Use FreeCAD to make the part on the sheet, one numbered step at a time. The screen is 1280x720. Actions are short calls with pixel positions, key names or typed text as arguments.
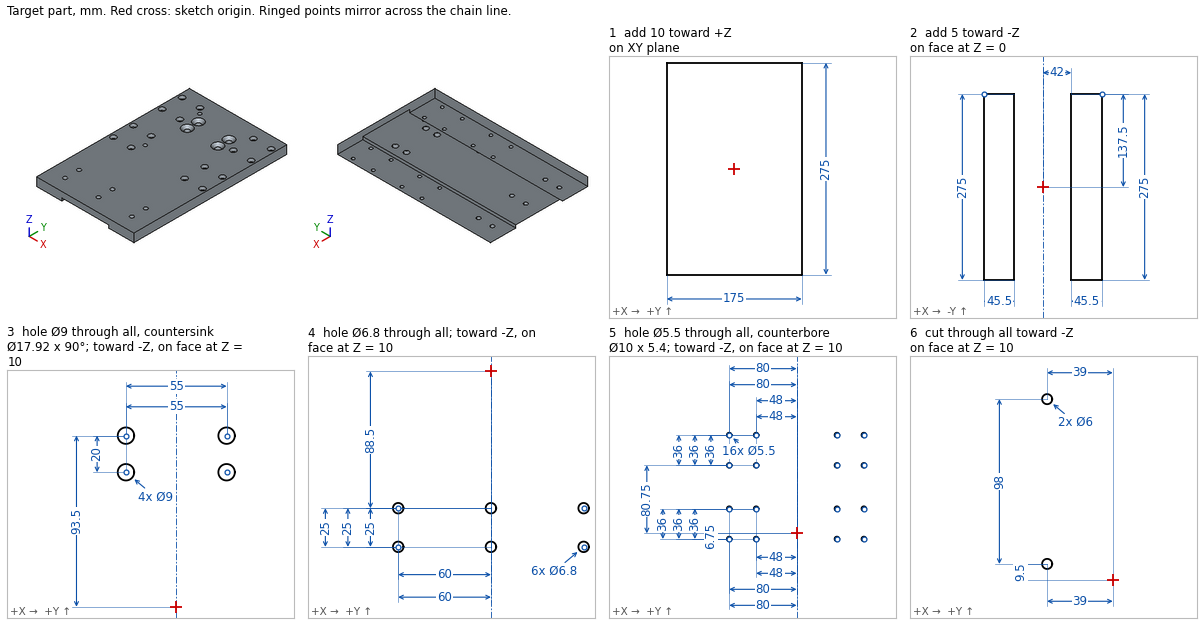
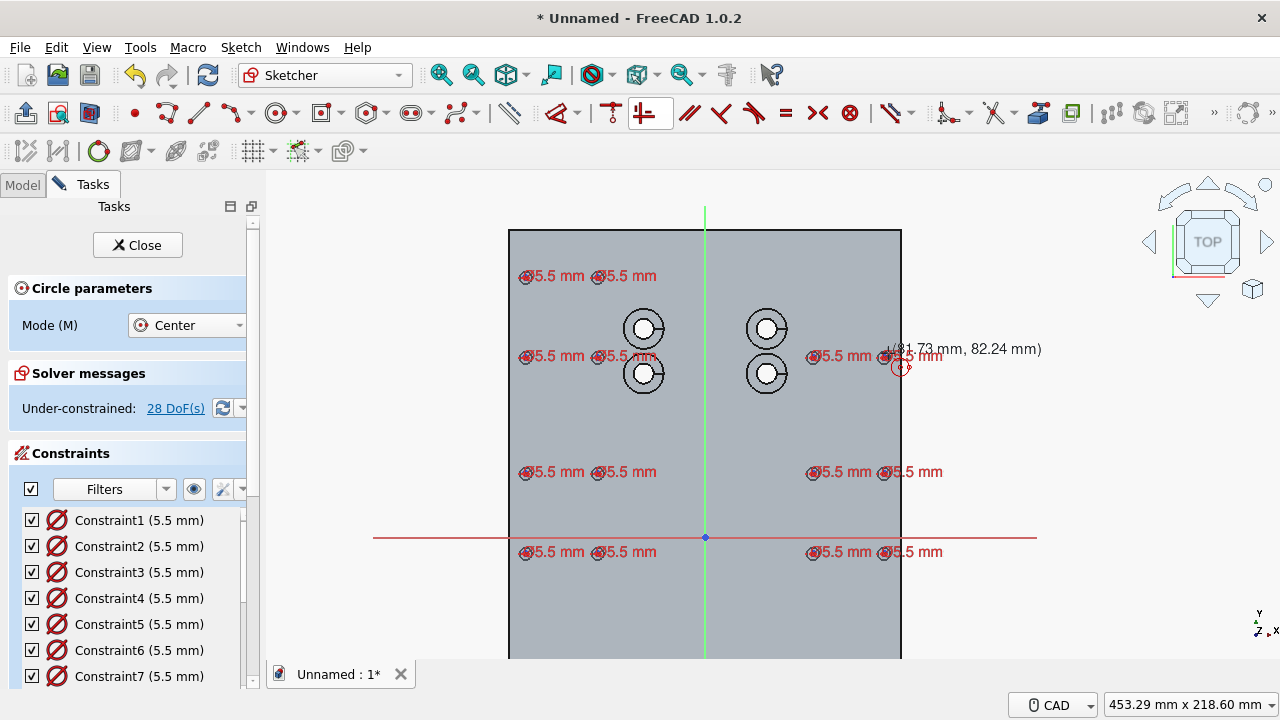
scroll(813, 277, up, 7)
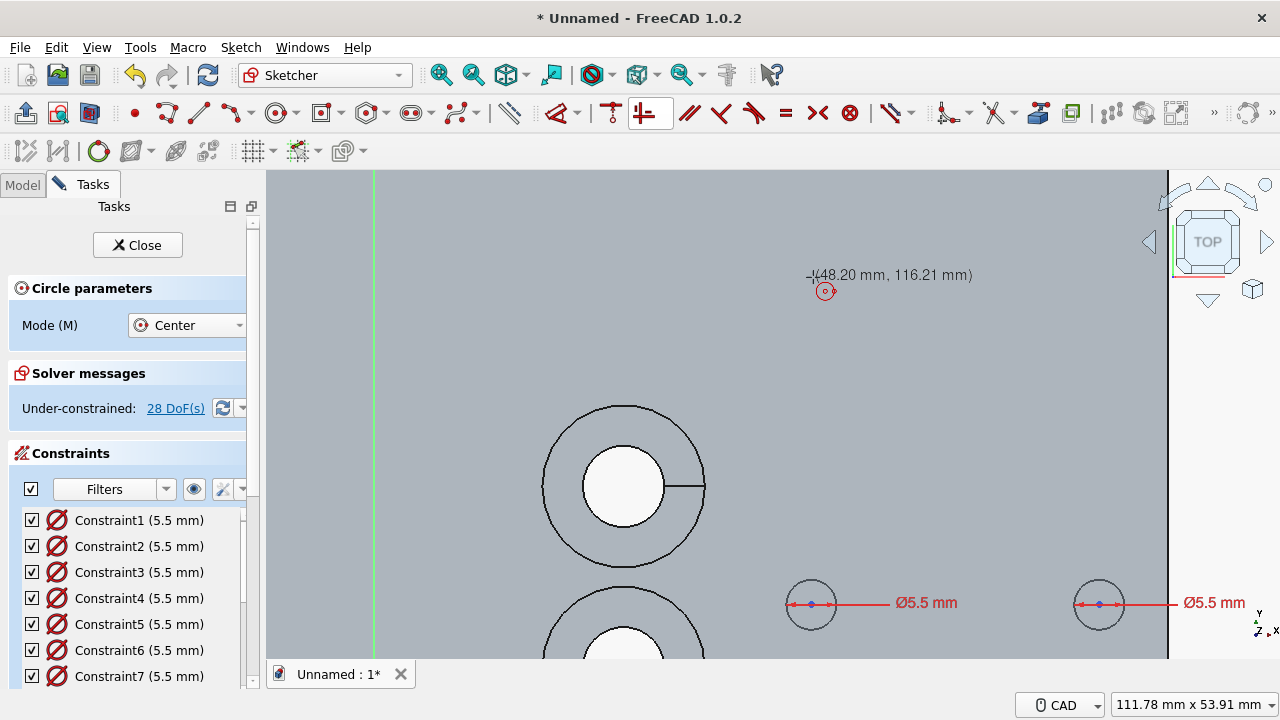
scroll(813, 277, down, 7)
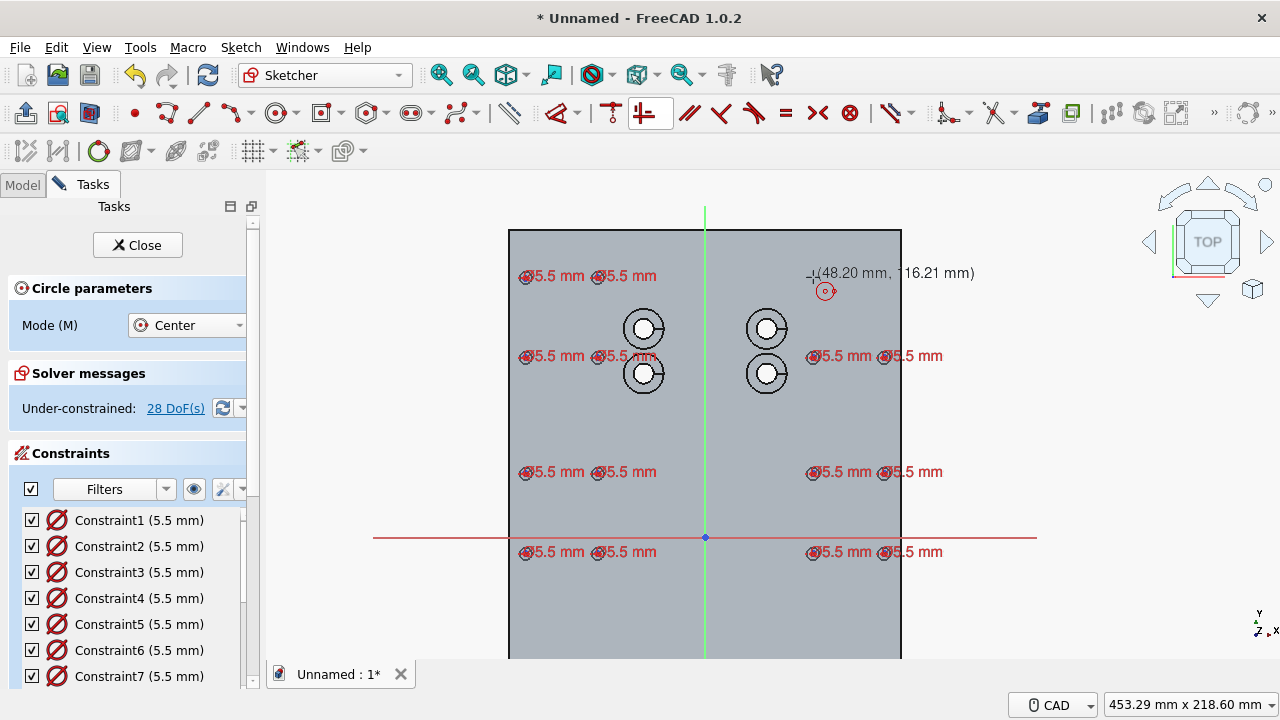
click(813, 277)
move(817, 272)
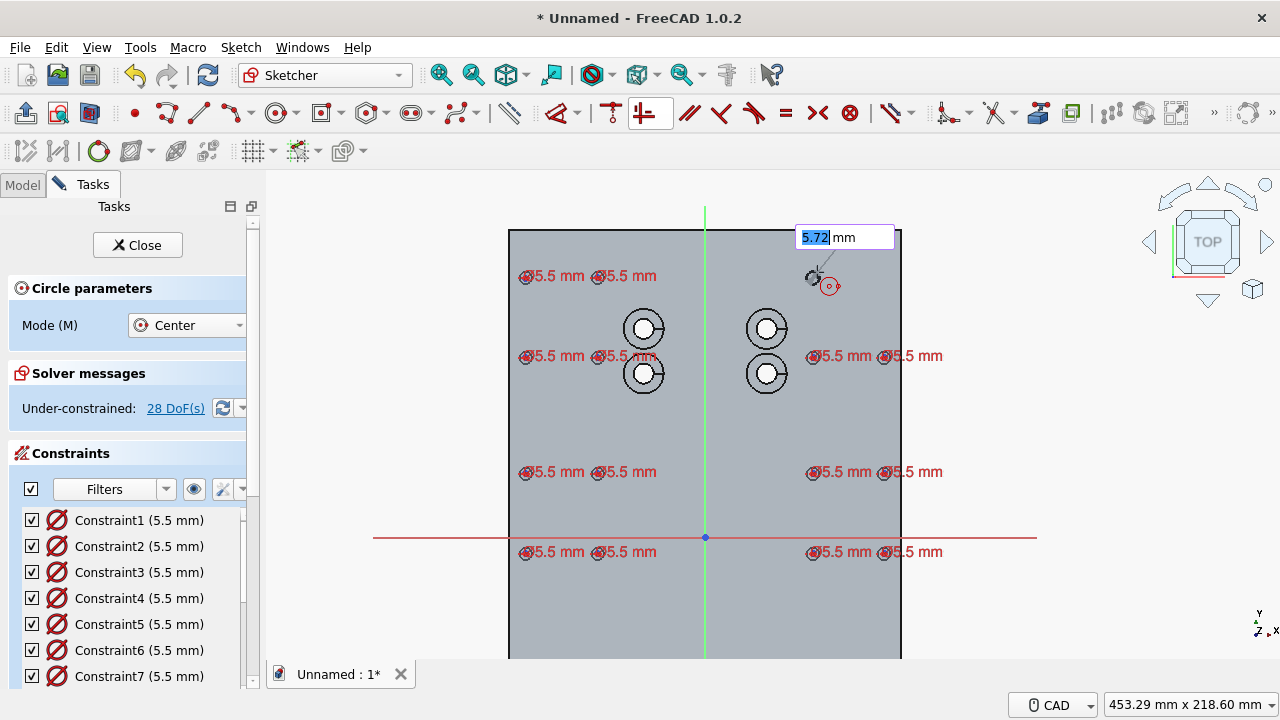
text(5.5)
key(Return)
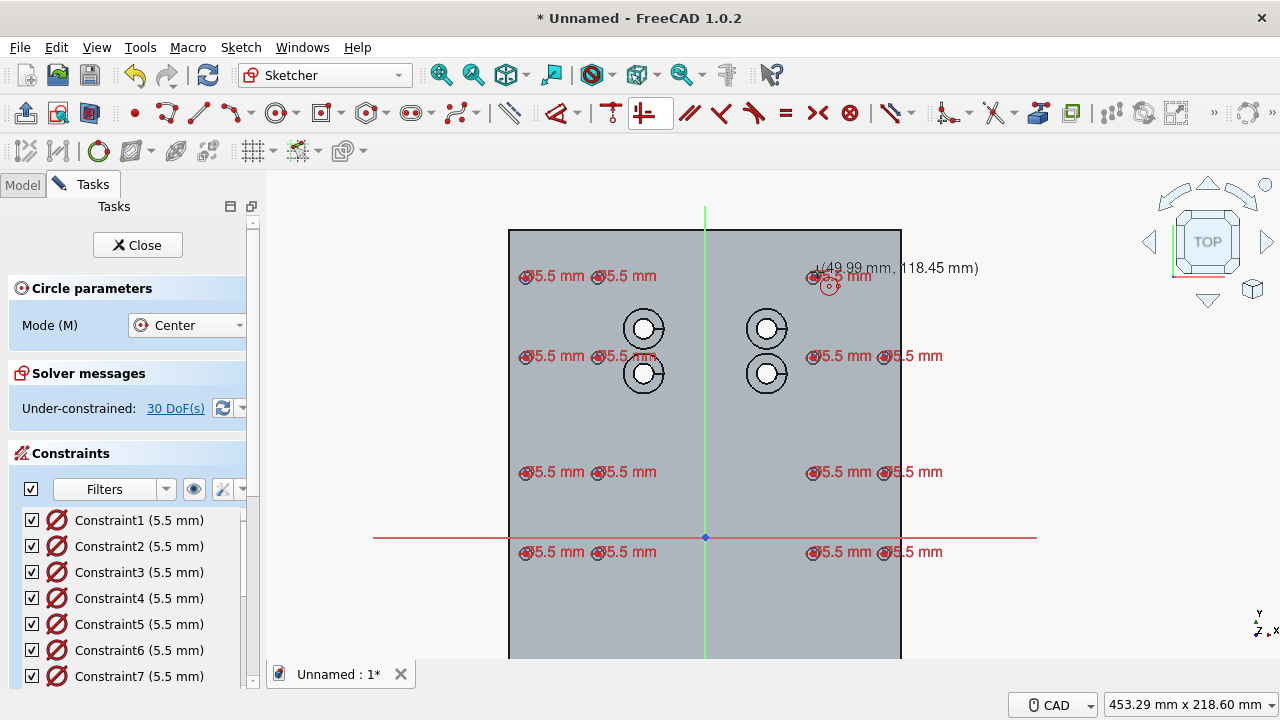
scroll(884, 277, up, 7)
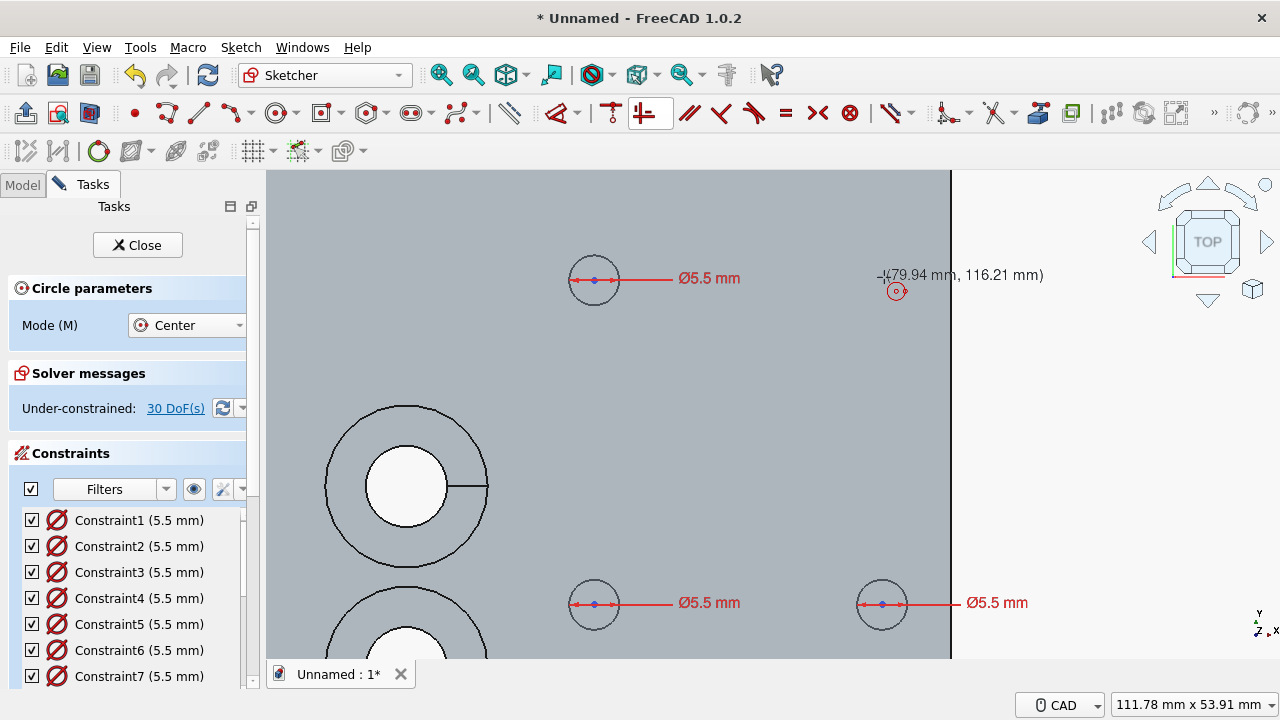
scroll(884, 277, down, 7)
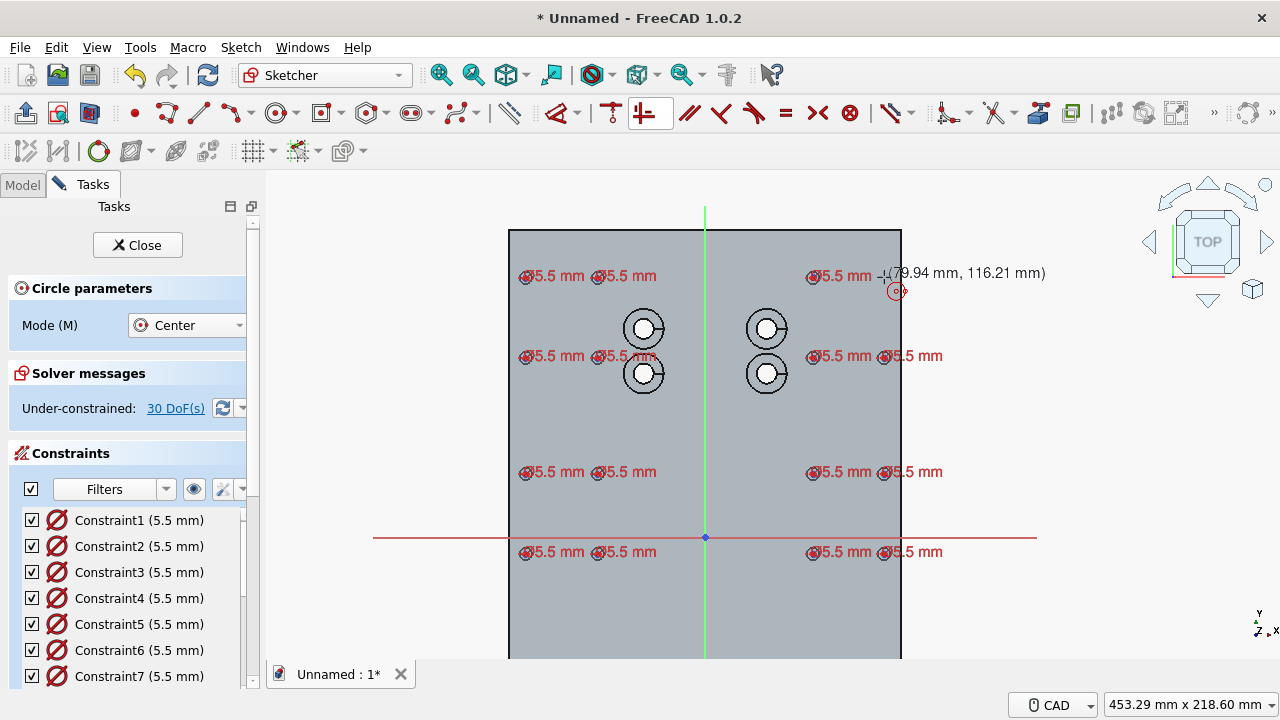
click(884, 277)
move(888, 272)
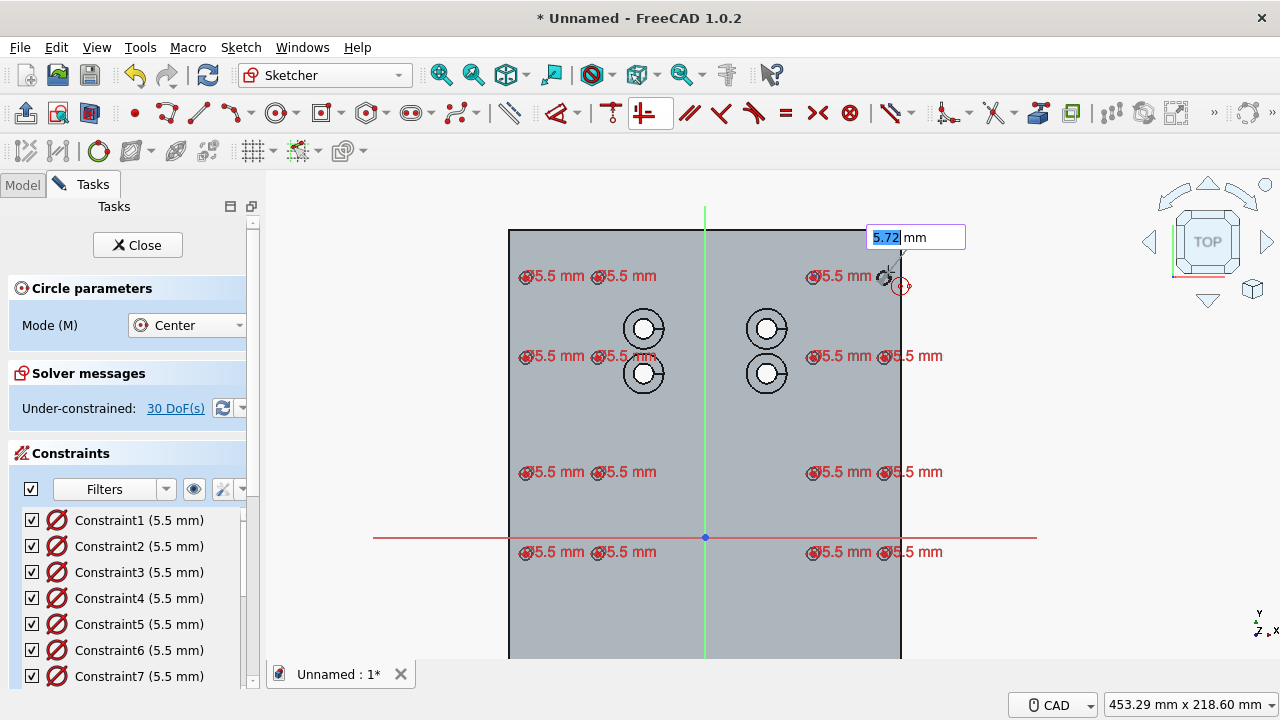
text(5.5)
key(Return)
key(Escape)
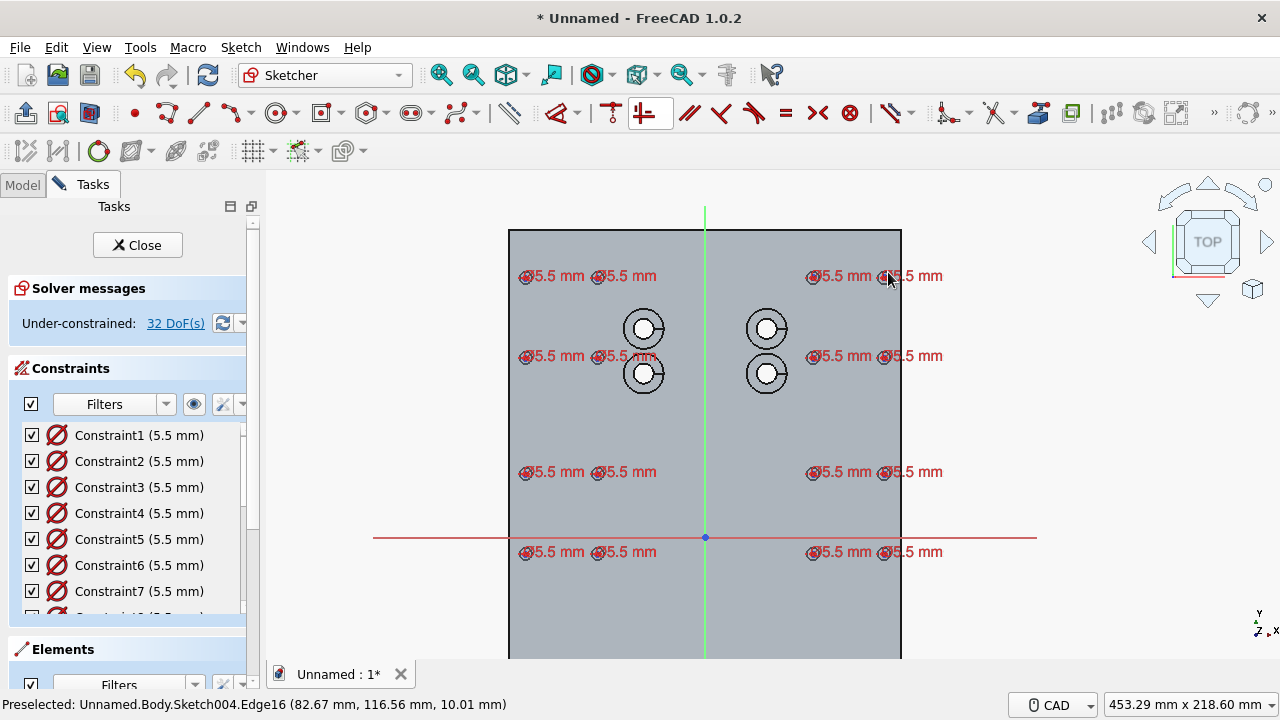
click(598, 554)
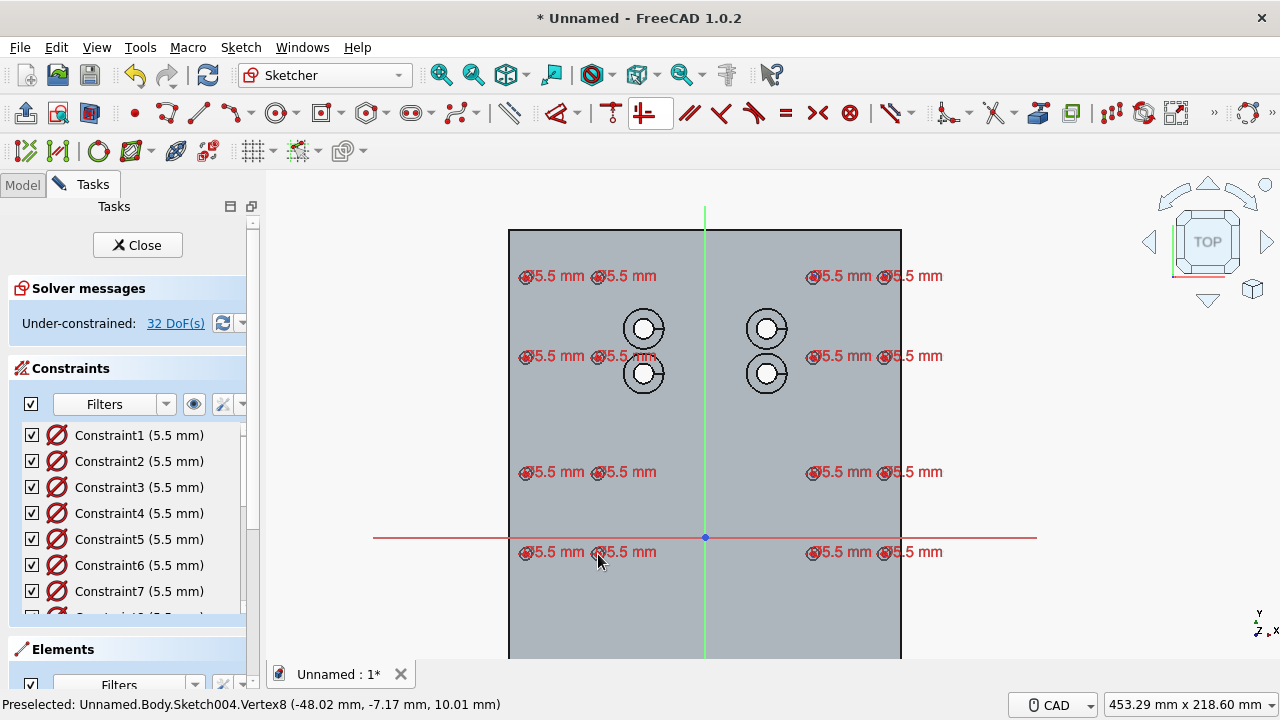
click(813, 554)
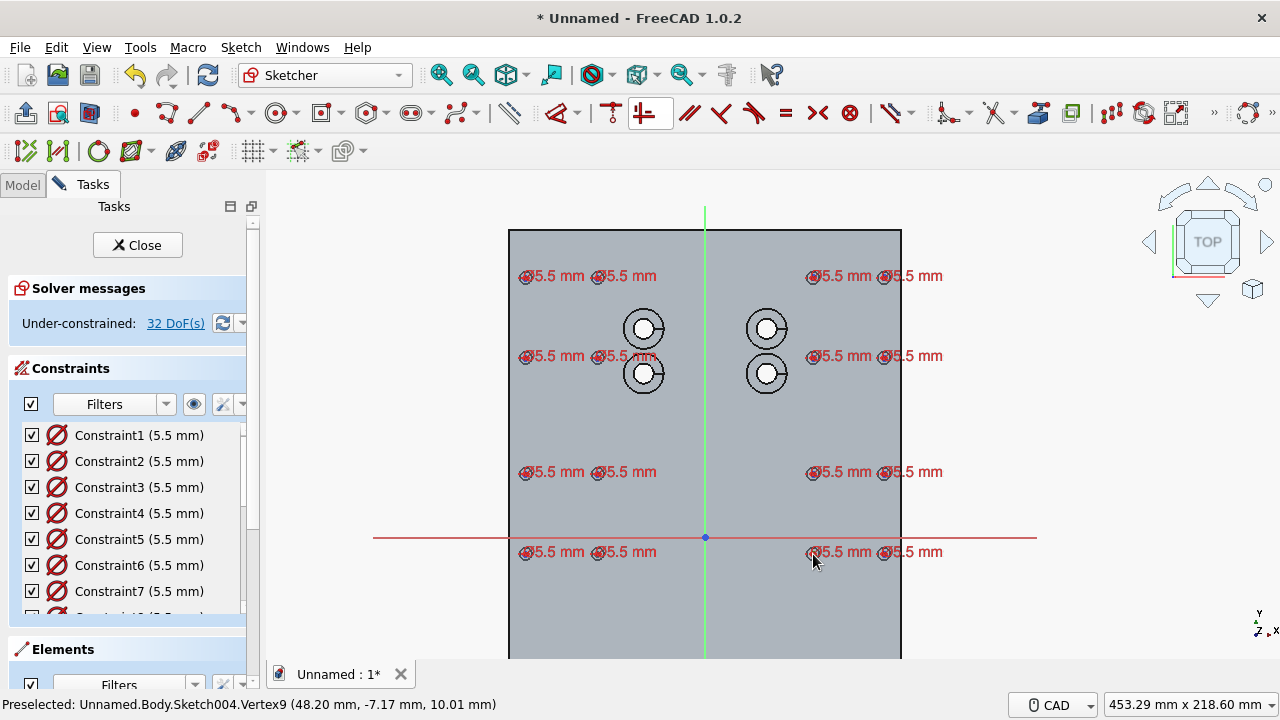
click(705, 600)